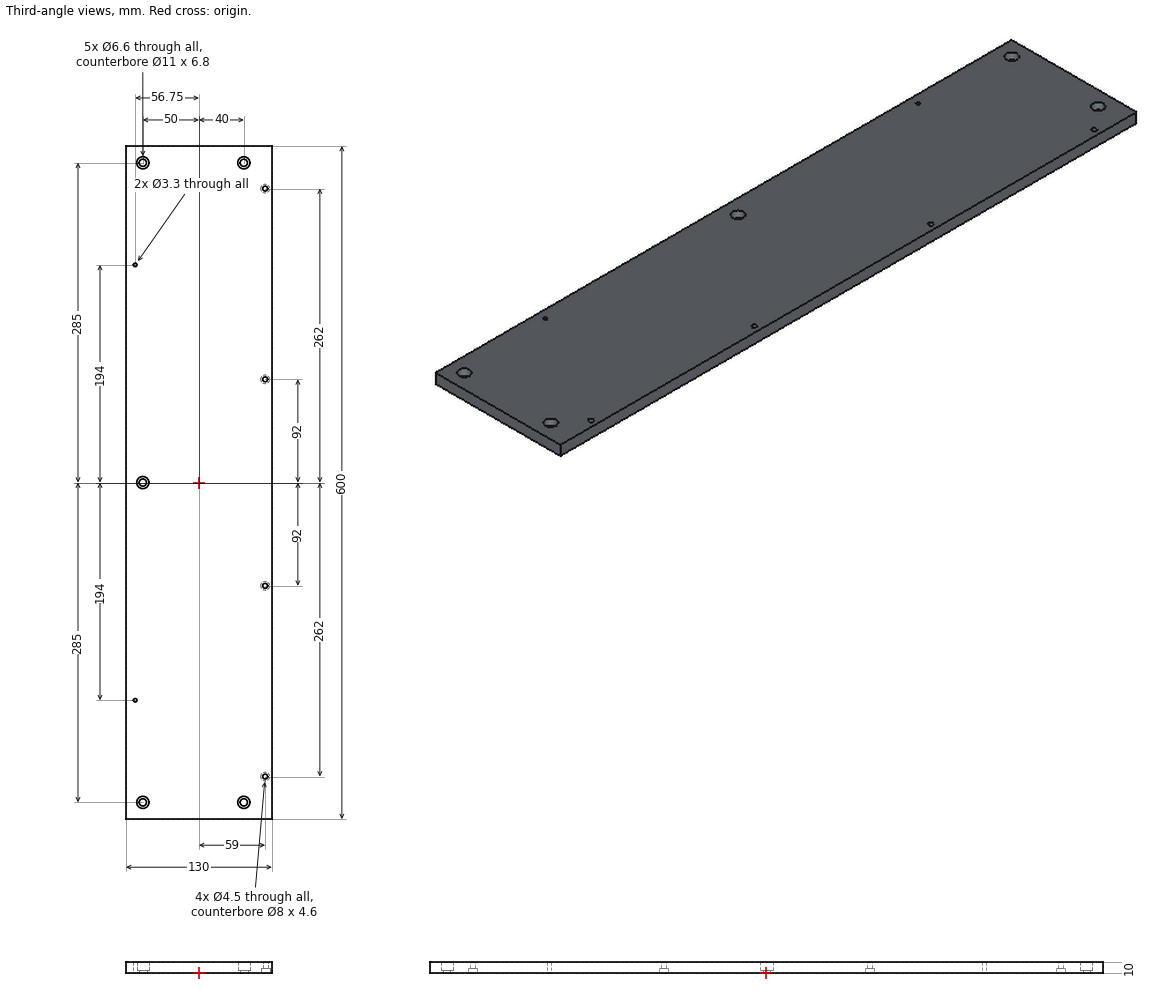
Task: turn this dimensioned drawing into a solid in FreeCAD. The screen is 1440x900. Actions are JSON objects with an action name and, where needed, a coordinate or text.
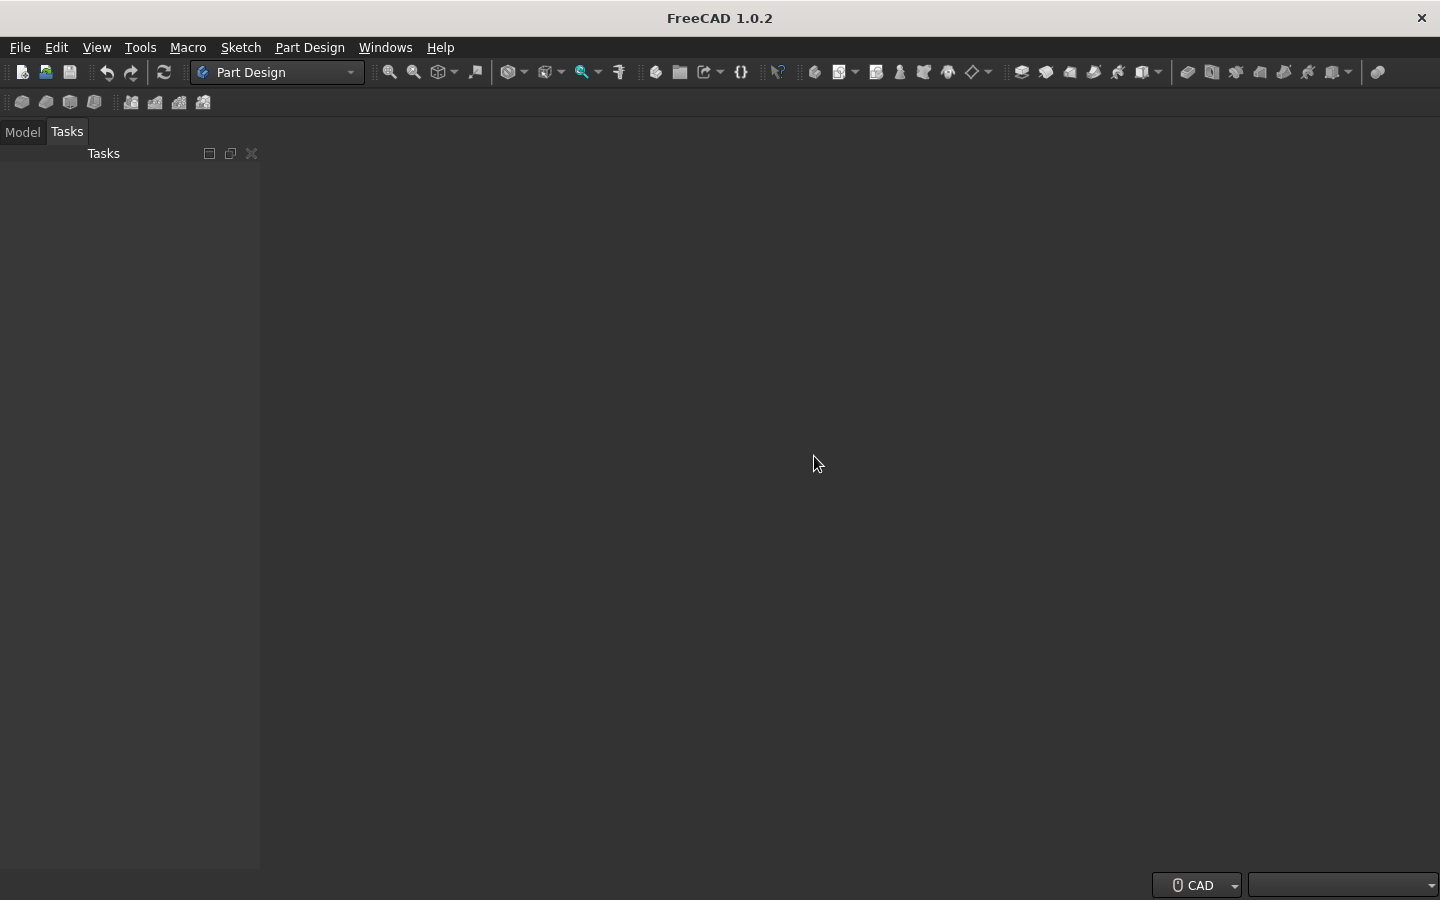
{"action": "key", "text": "ctrl+n"}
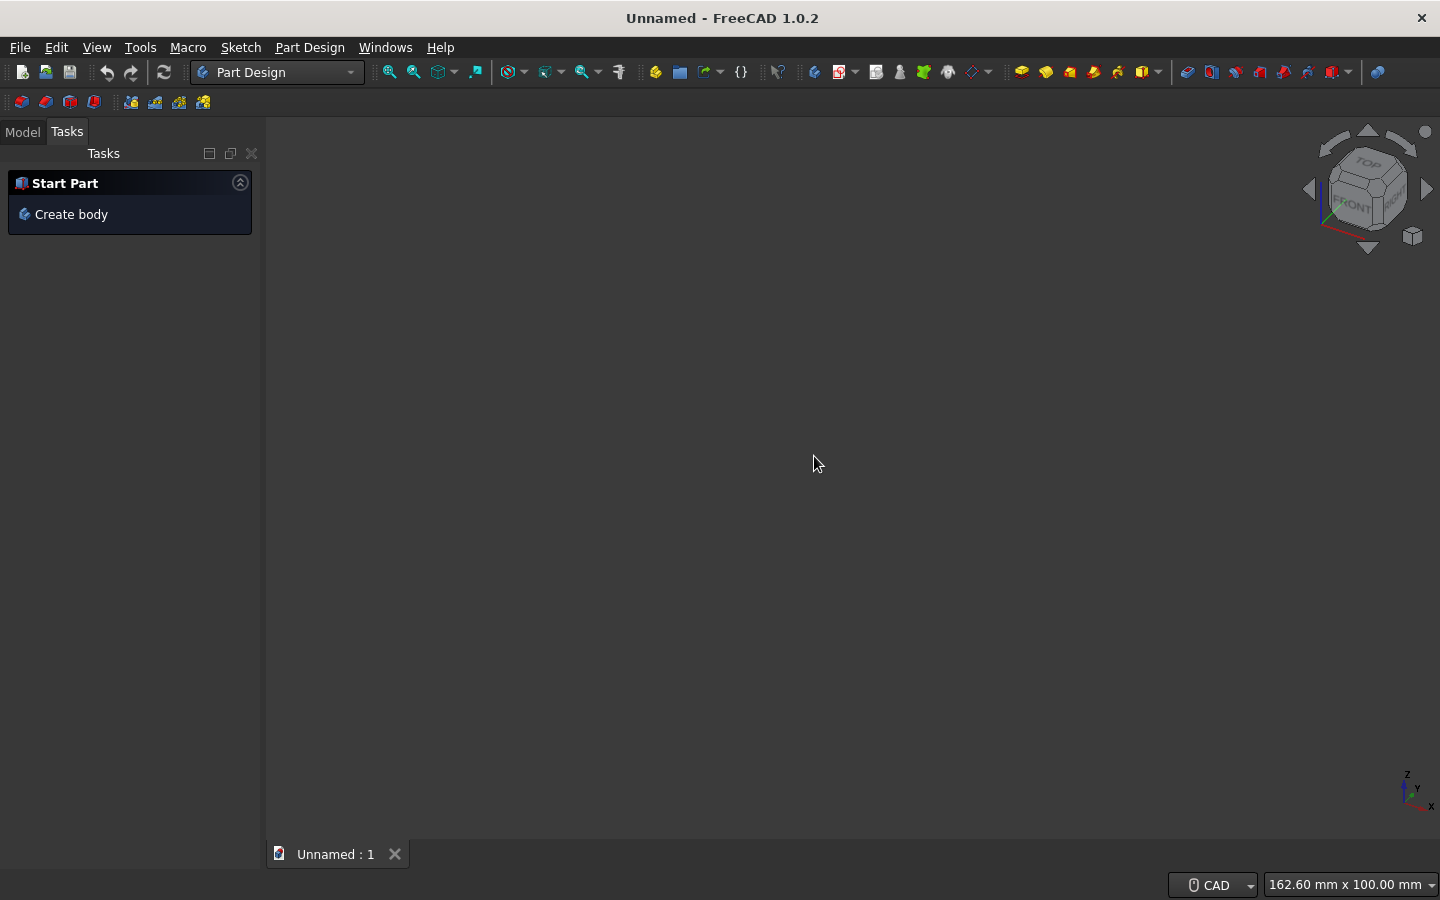
{"action": "left_click", "coordinate": [840, 72]}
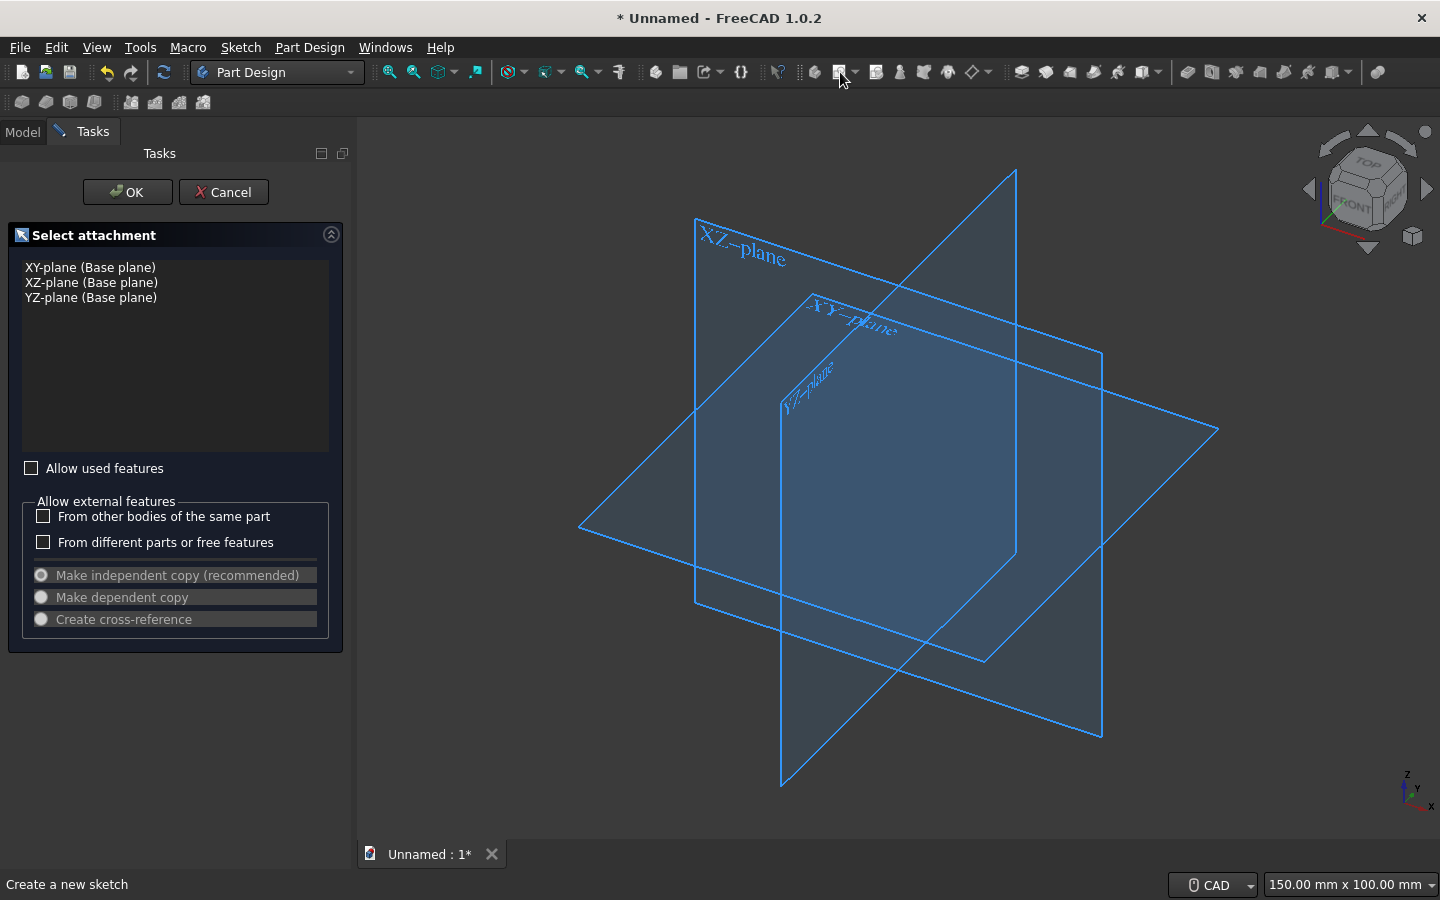
{"action": "left_click", "coordinate": [82, 268]}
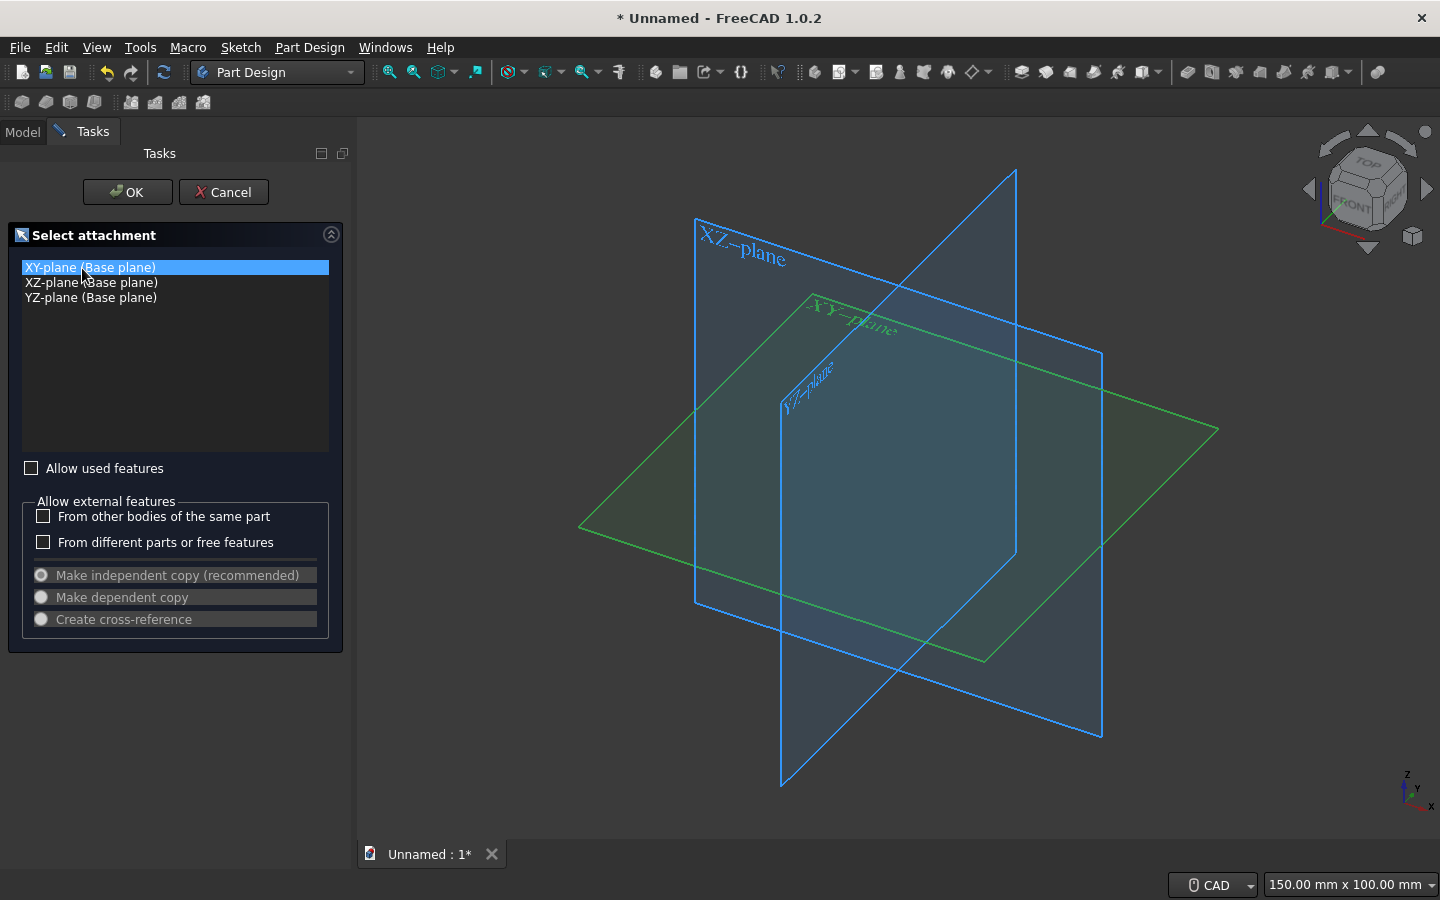
{"action": "left_click", "coordinate": [128, 192]}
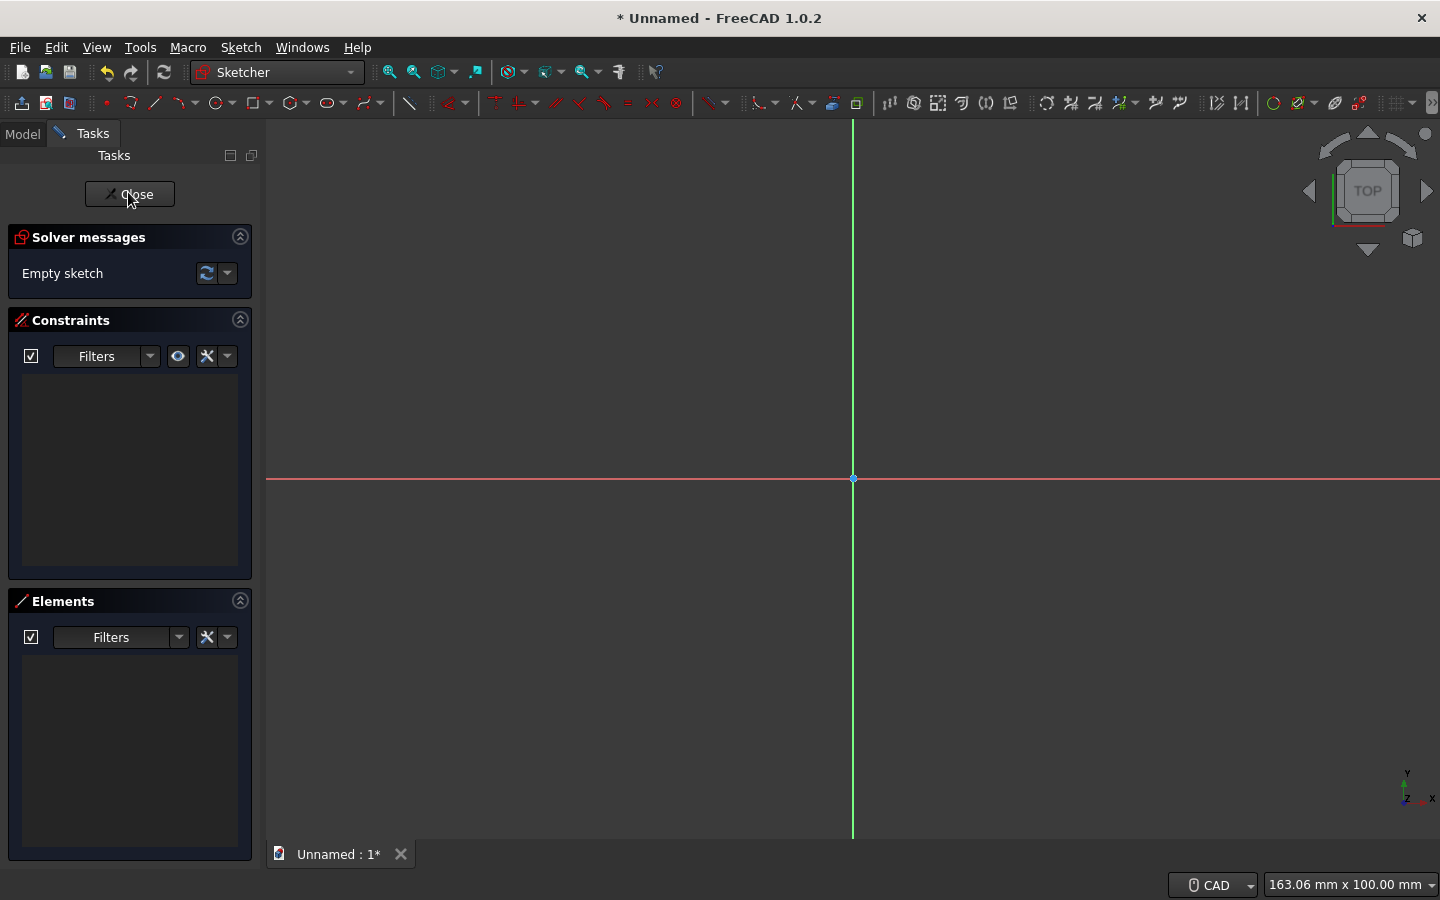
{"action": "scroll", "coordinate": [776, 479], "scroll_direction": "down", "scroll_amount": 11}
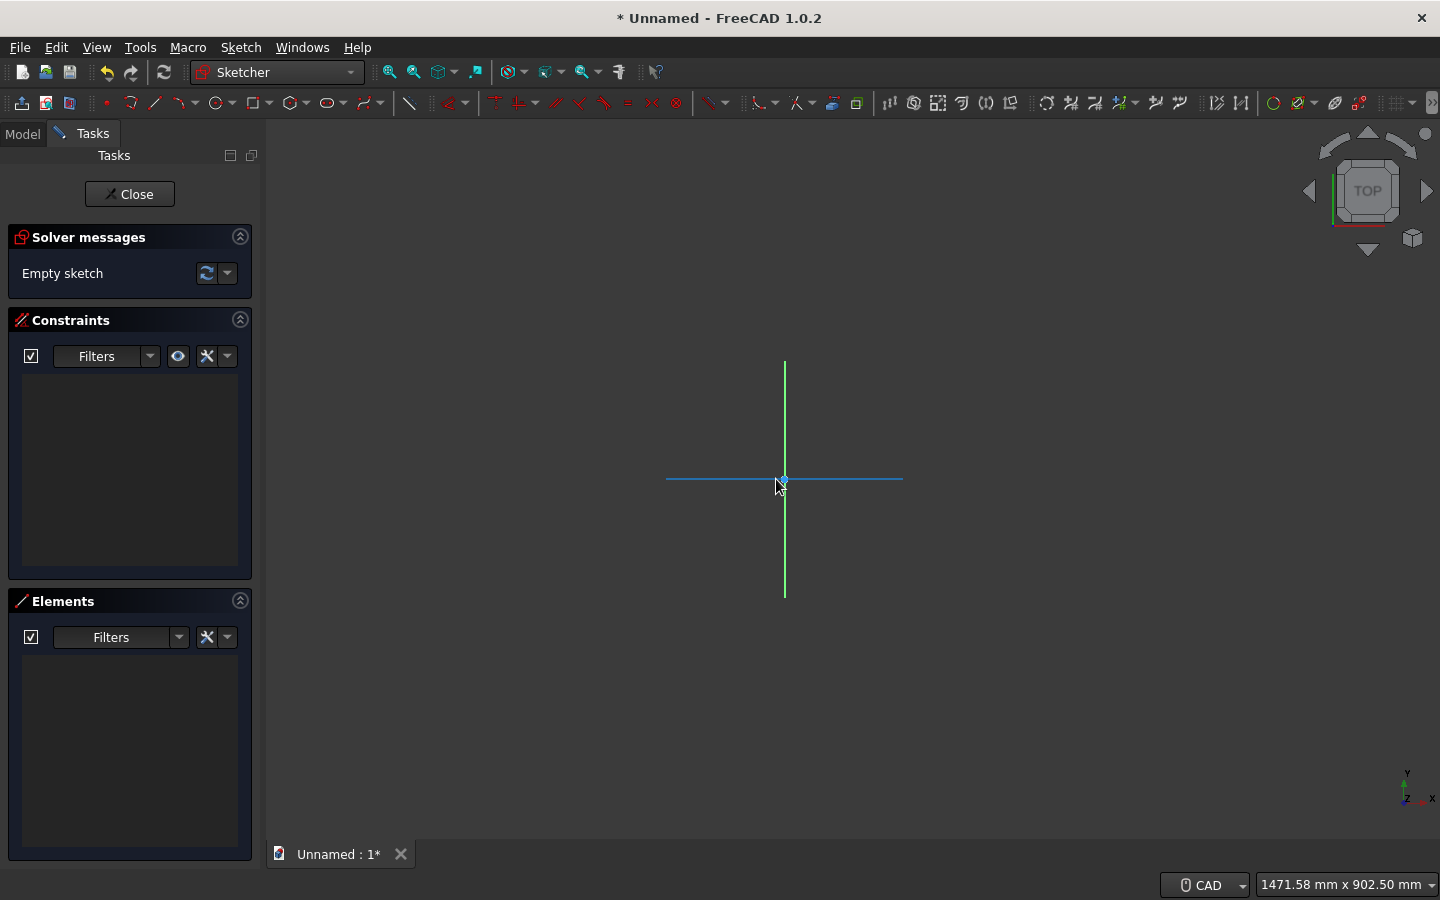
{"action": "key", "text": "g v"}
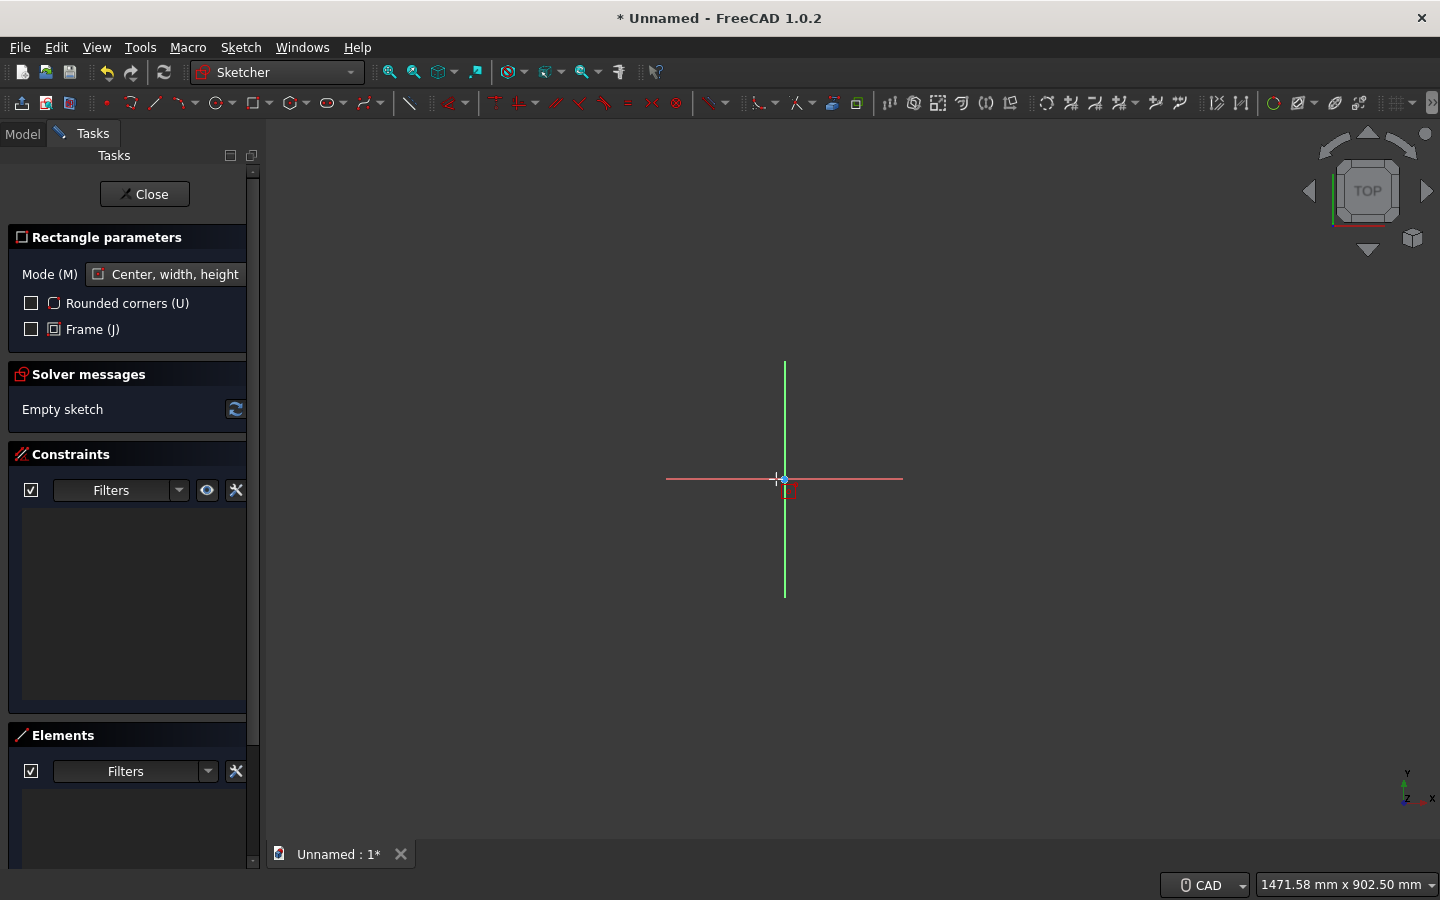
{"action": "left_click", "coordinate": [785, 479]}
{"action": "mouse_move", "coordinate": [837, 240]}